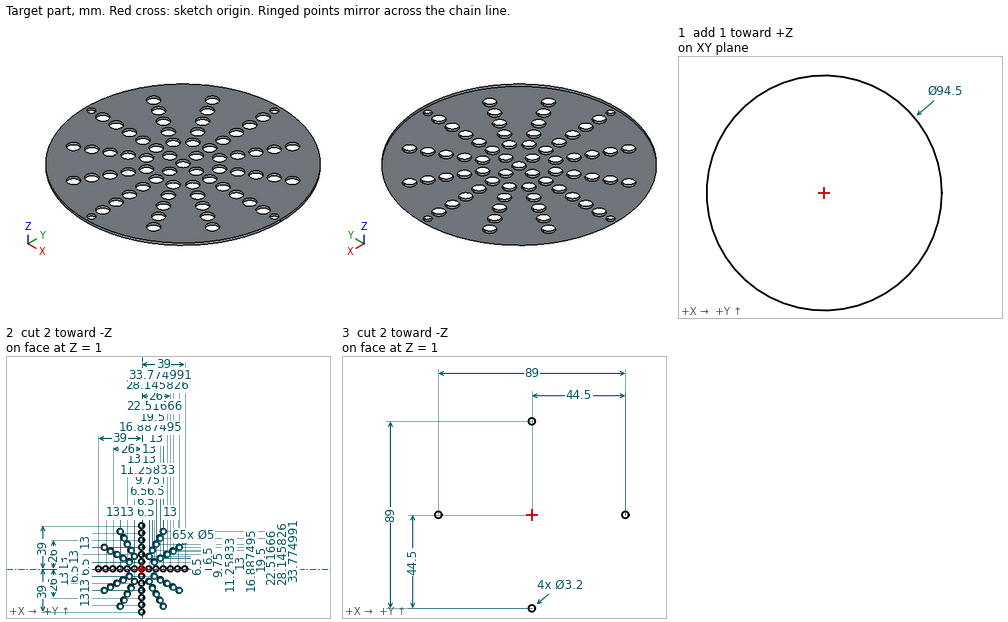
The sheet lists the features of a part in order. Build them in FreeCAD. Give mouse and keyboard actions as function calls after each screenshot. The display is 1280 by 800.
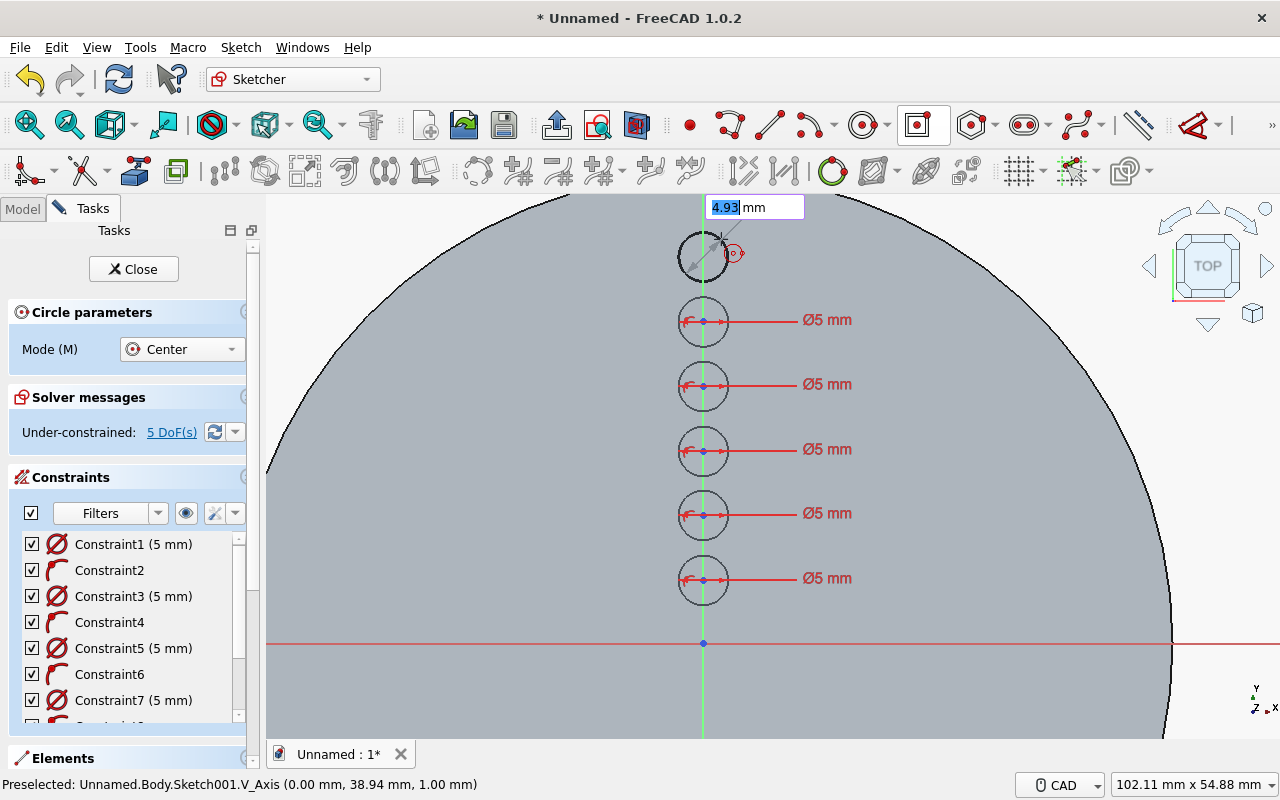
text(5)
key(Return)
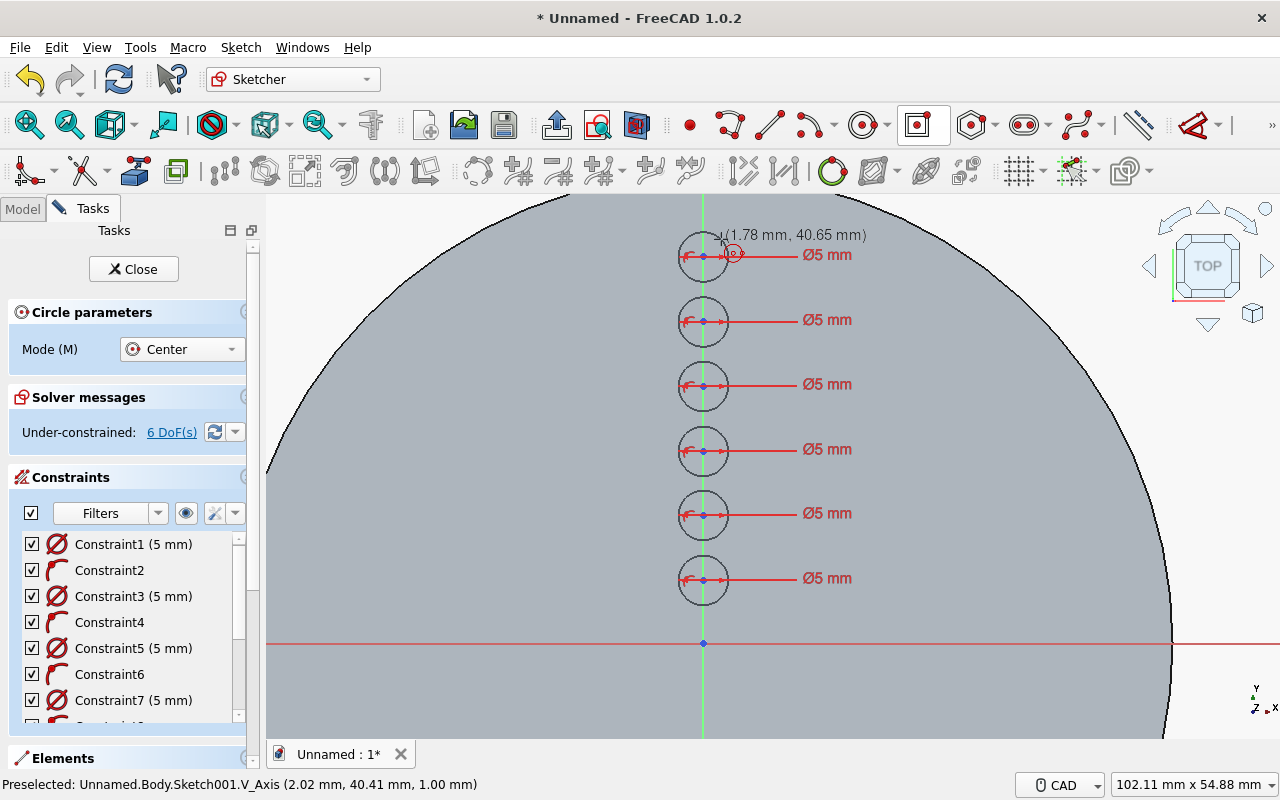
click(703, 644)
move(721, 626)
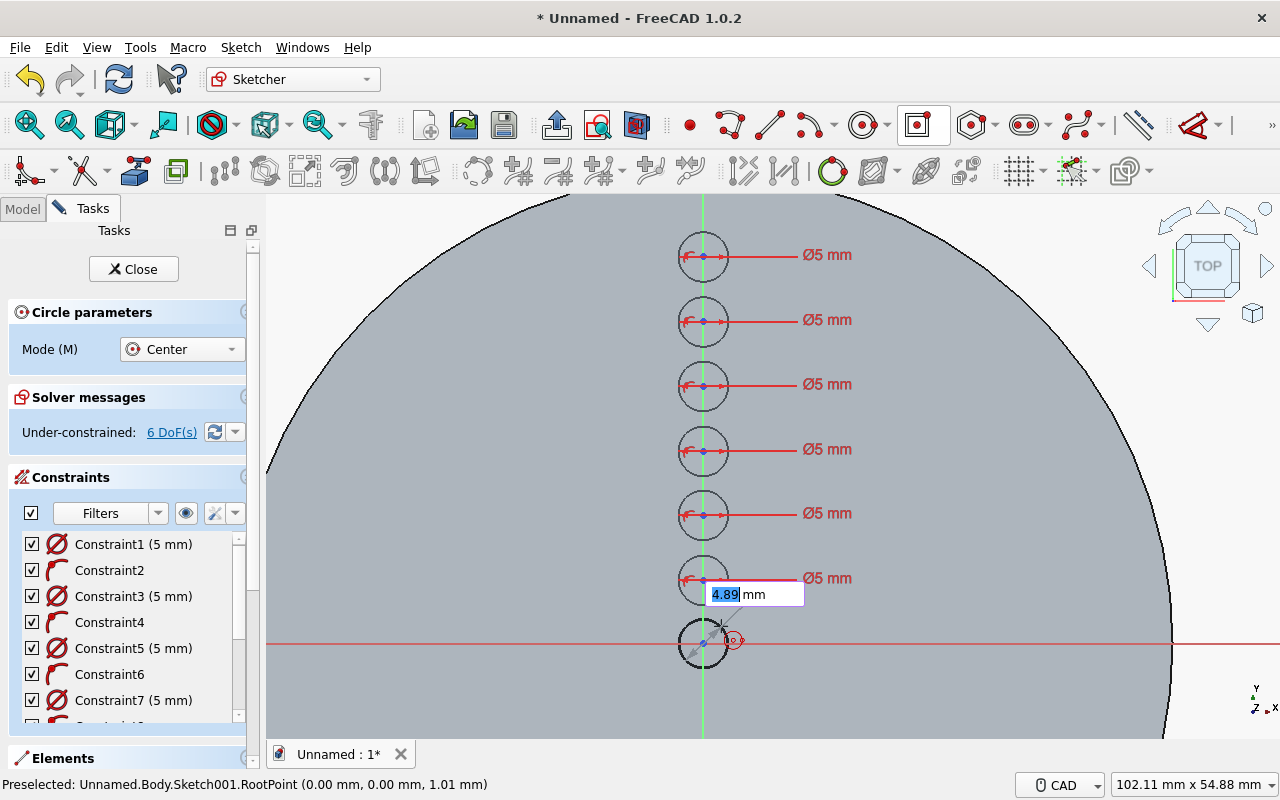
text(5)
key(Return)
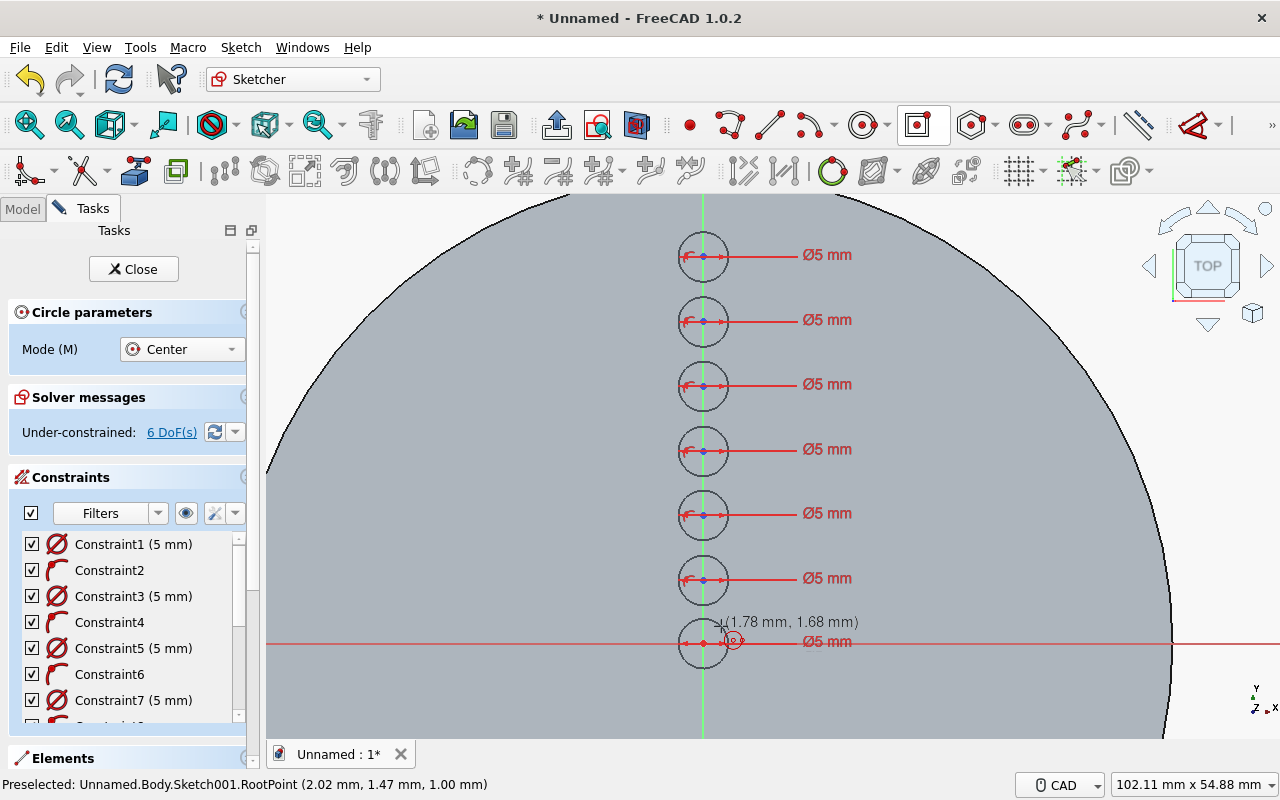
click(897, 308)
move(915, 291)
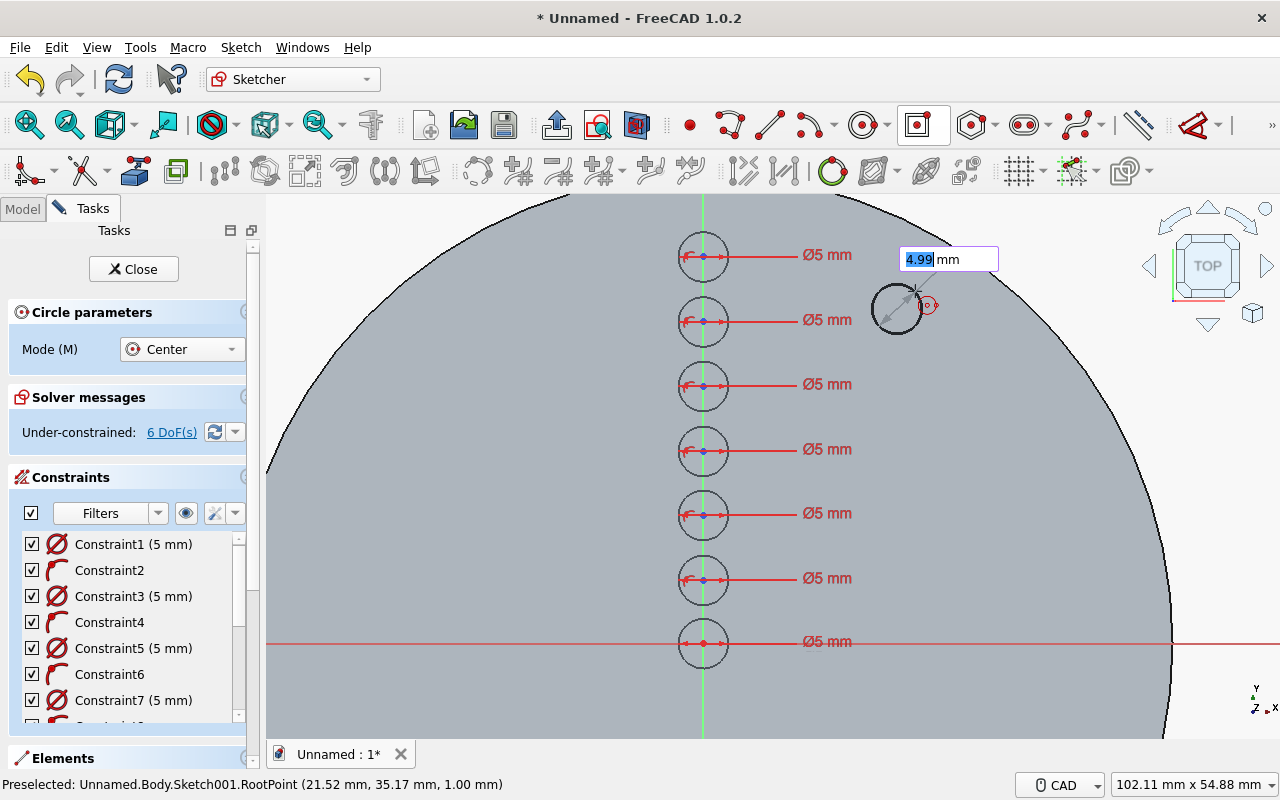
text(5)
key(Return)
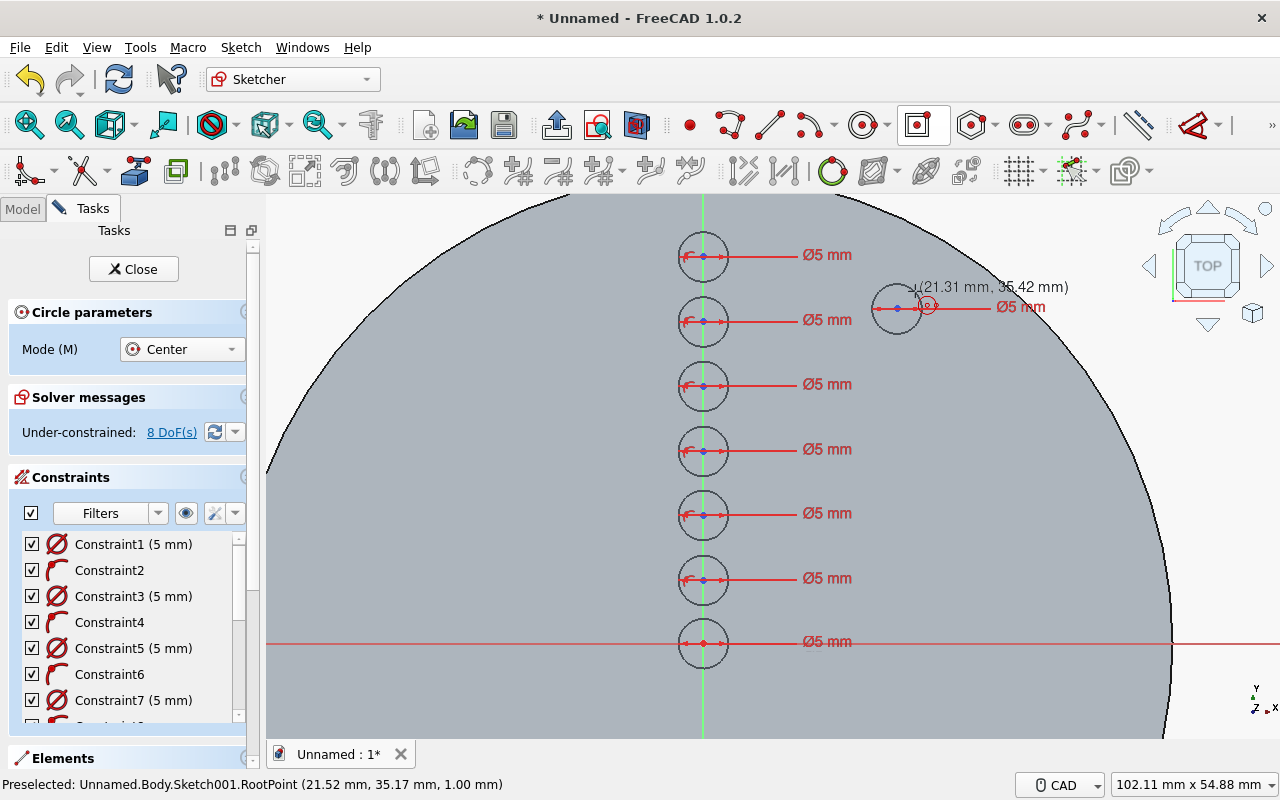
click(865, 364)
move(882, 347)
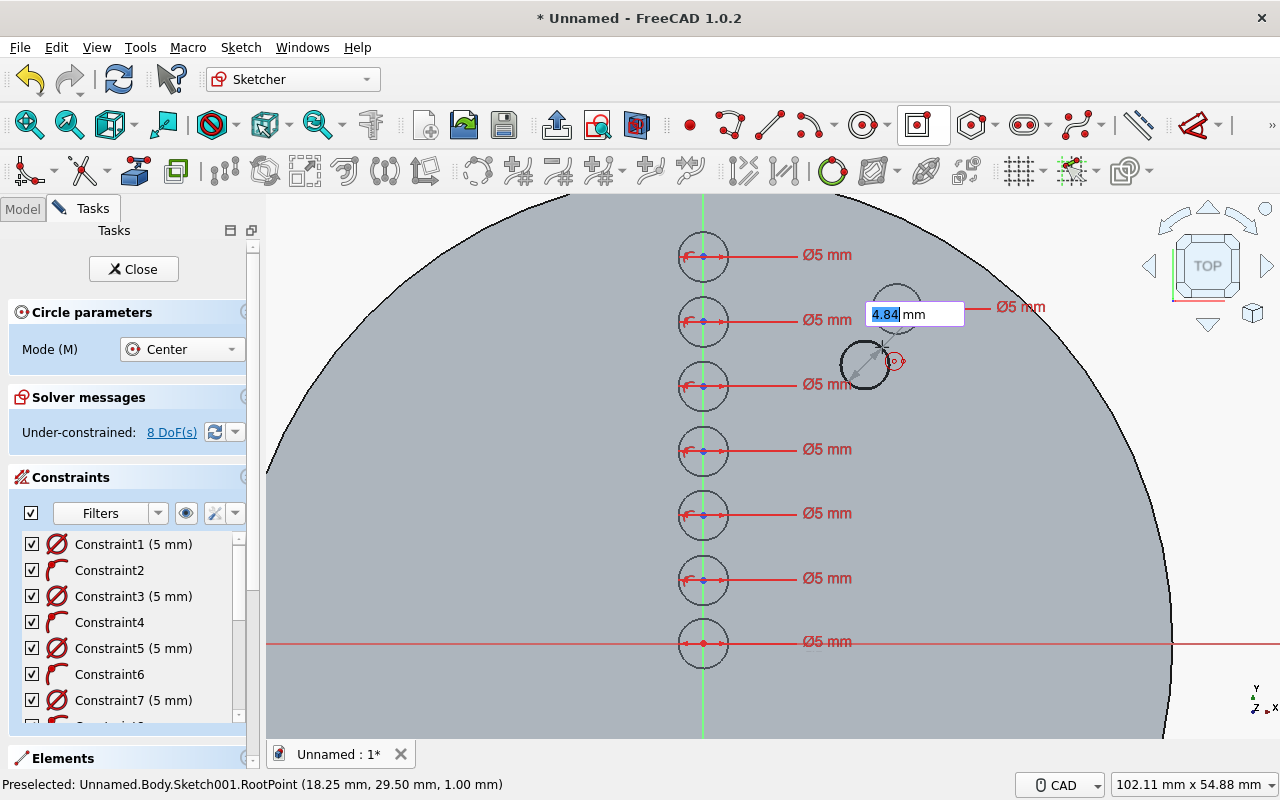
text(5)
key(Return)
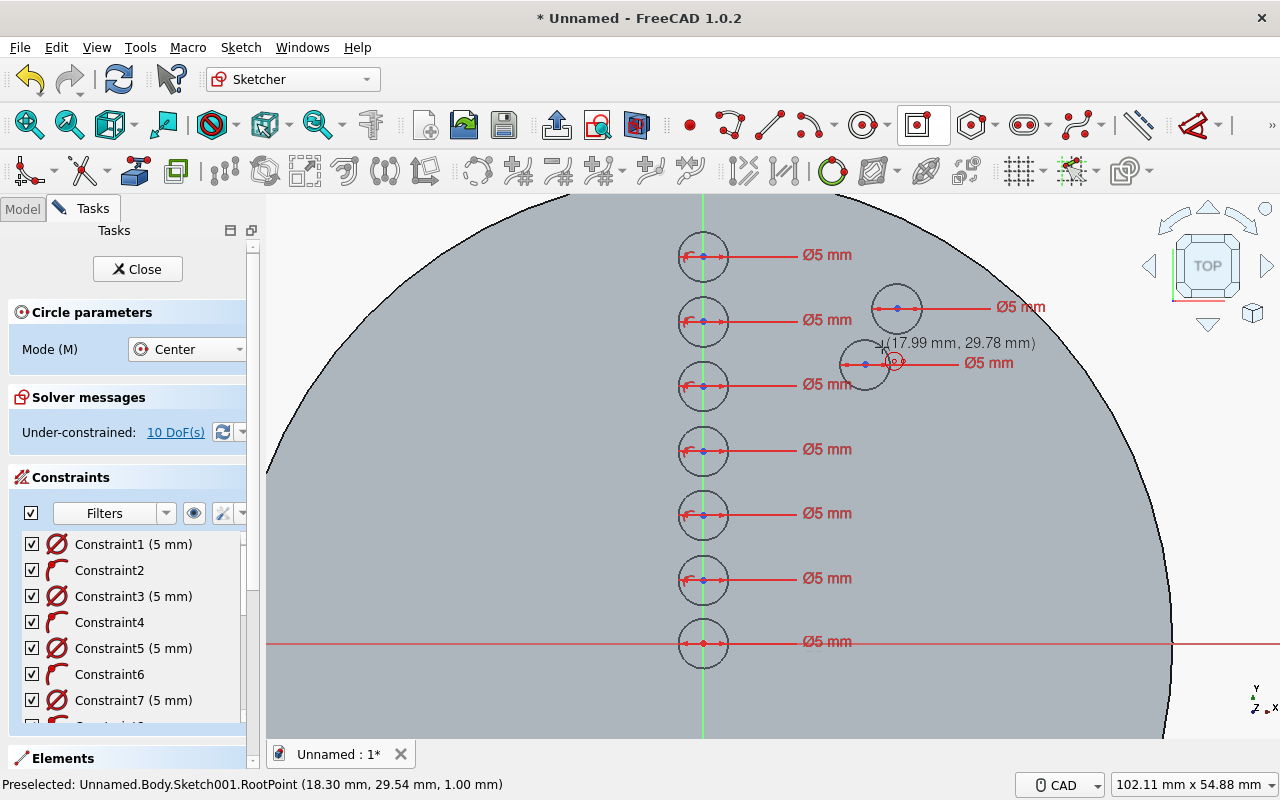
click(832, 420)
move(850, 403)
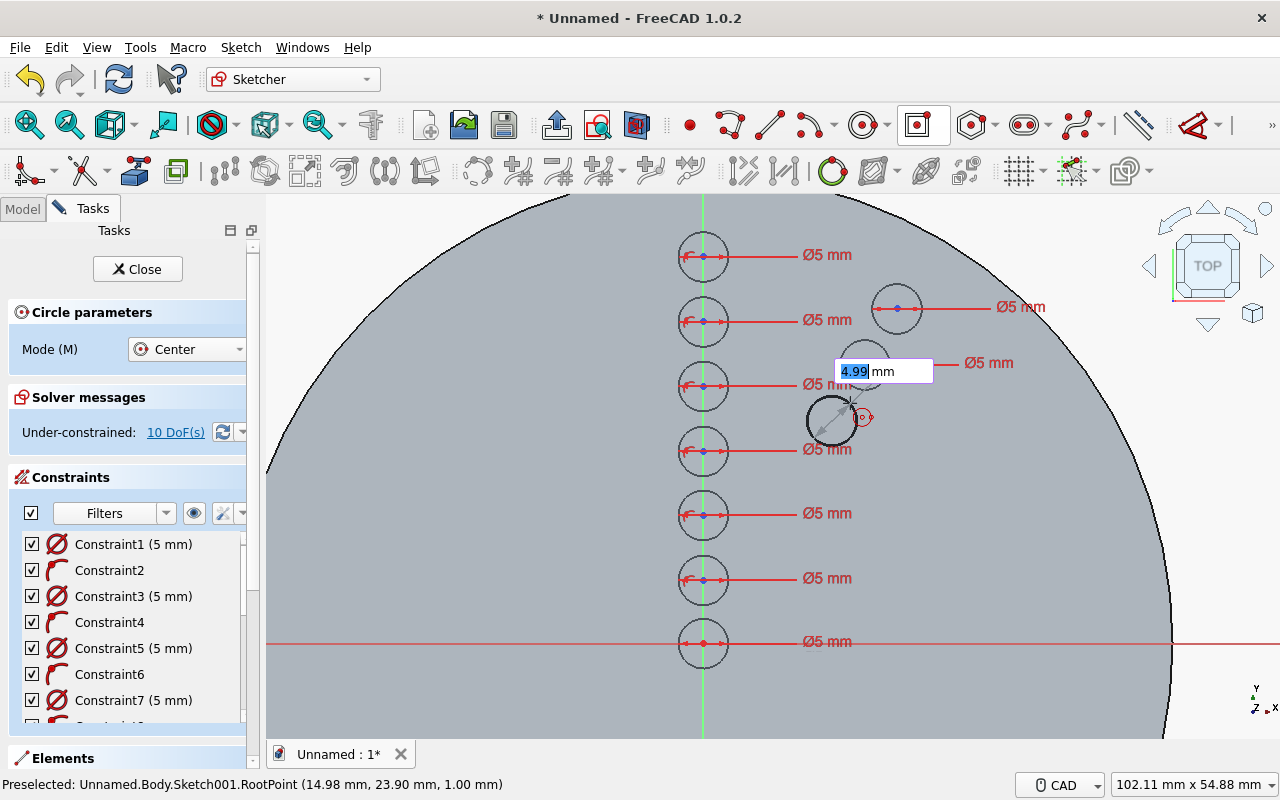
text(5)
key(Return)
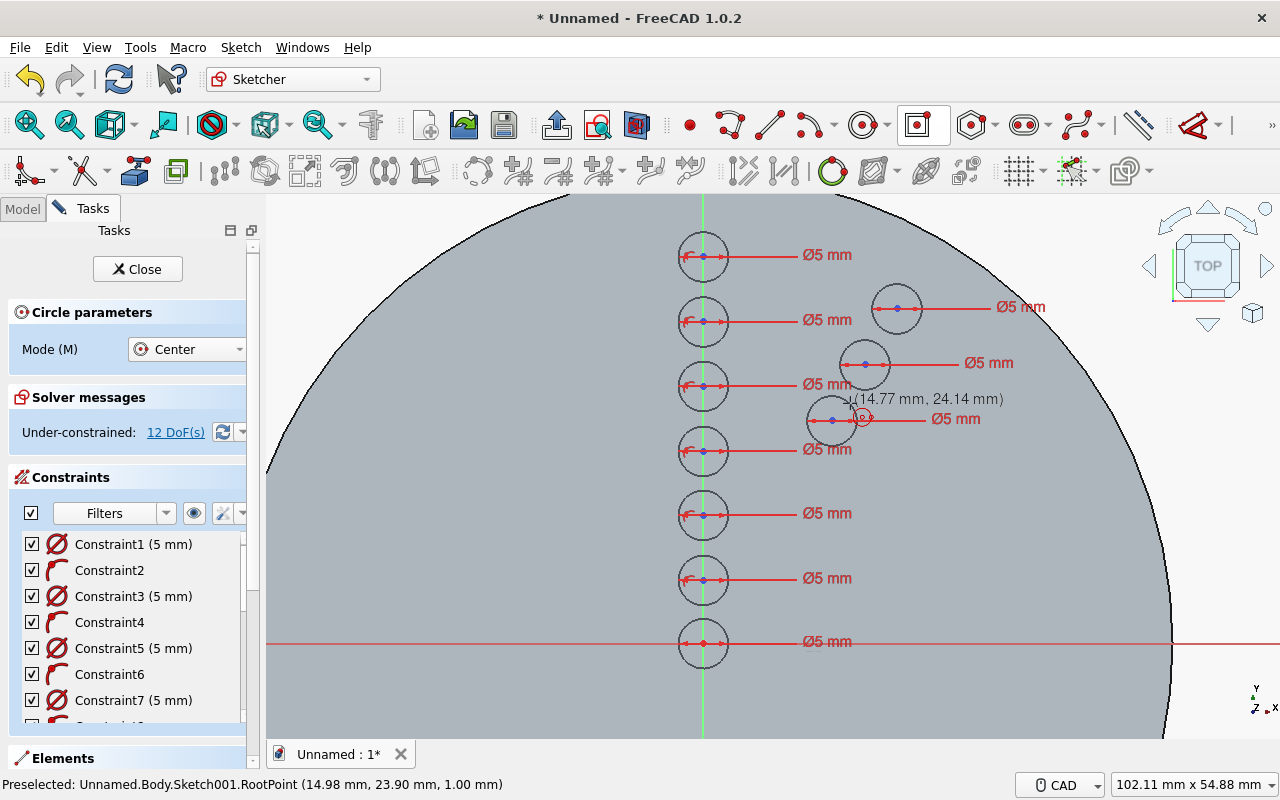
click(800, 476)
move(818, 458)